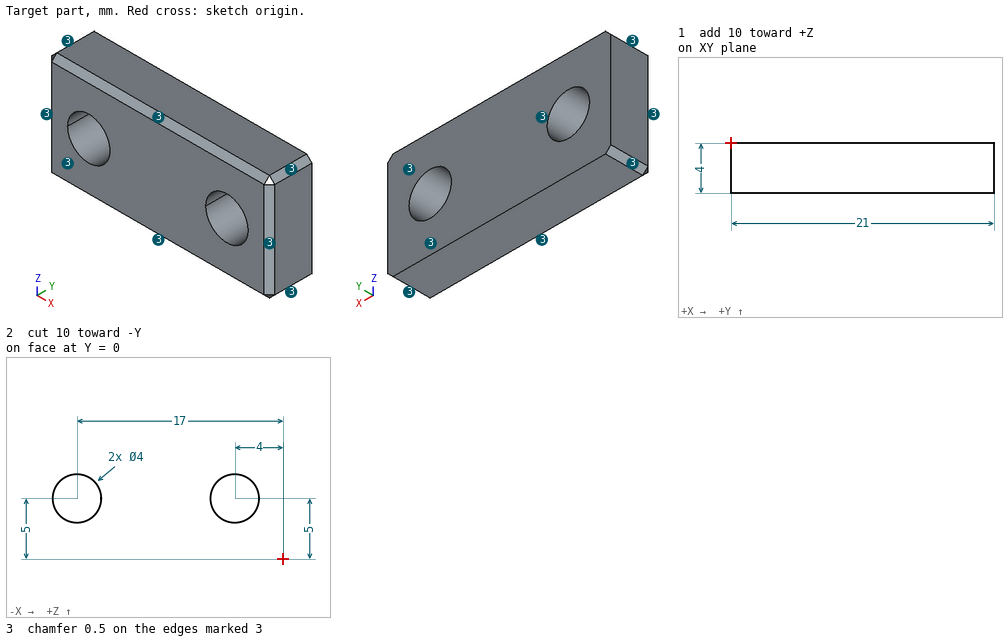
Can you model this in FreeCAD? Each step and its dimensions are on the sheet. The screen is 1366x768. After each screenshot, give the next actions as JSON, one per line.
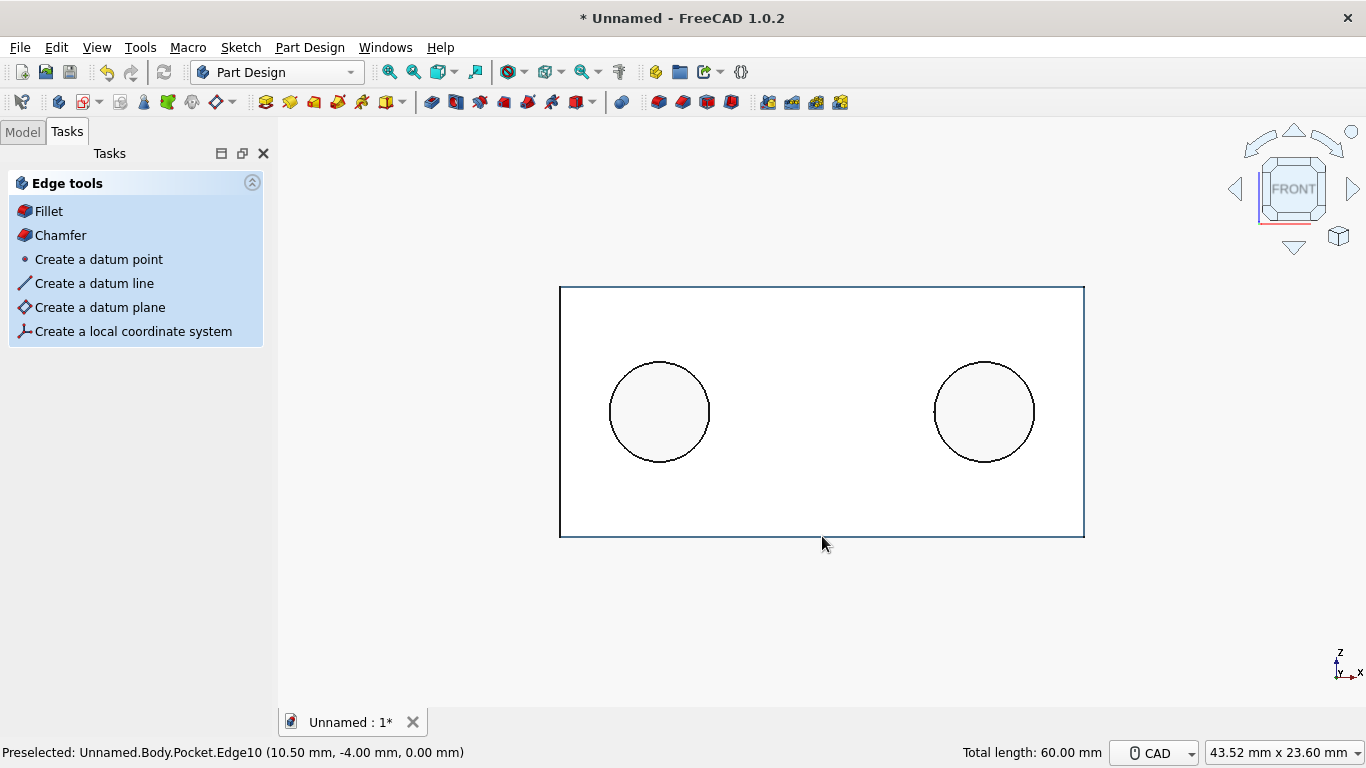
{"action": "left_click", "coordinate": [560, 411], "text": "ctrl"}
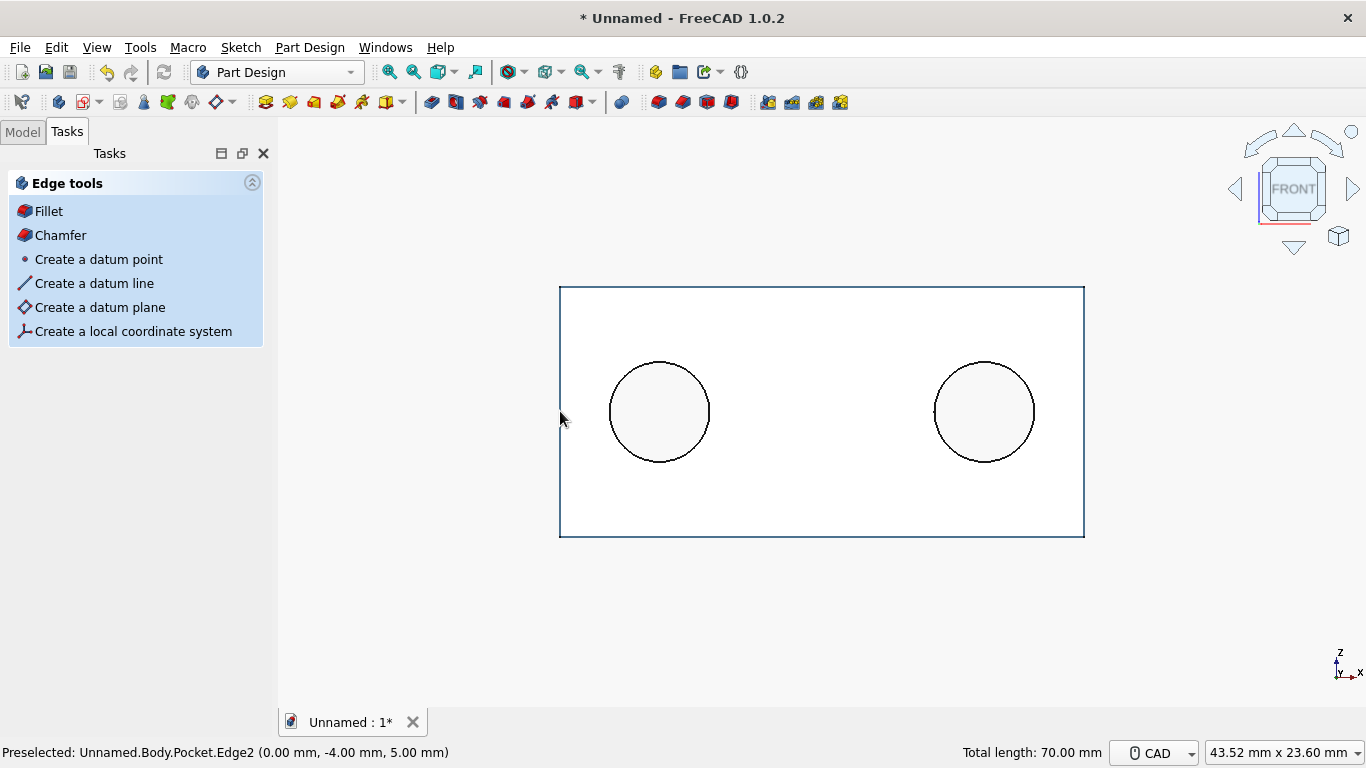
{"action": "key", "text": "3"}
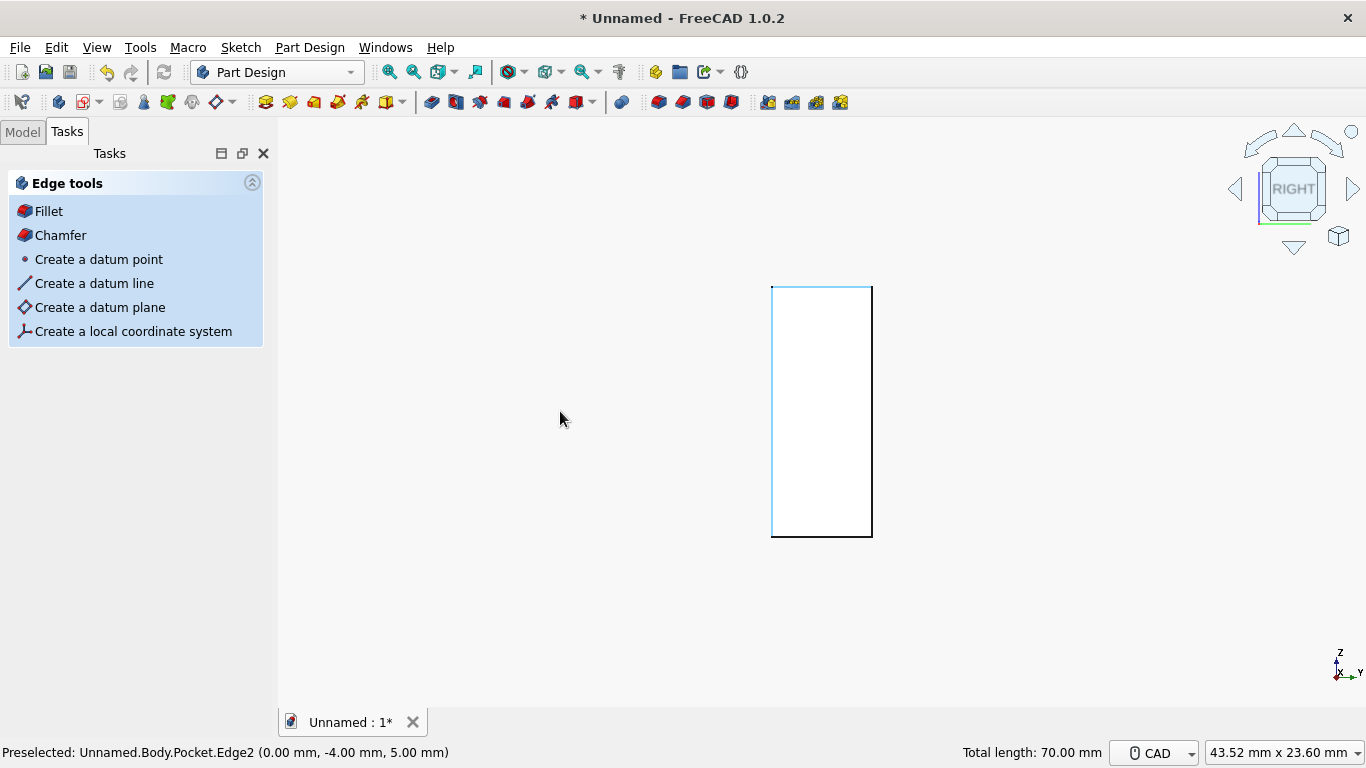
{"action": "left_click", "coordinate": [390, 72]}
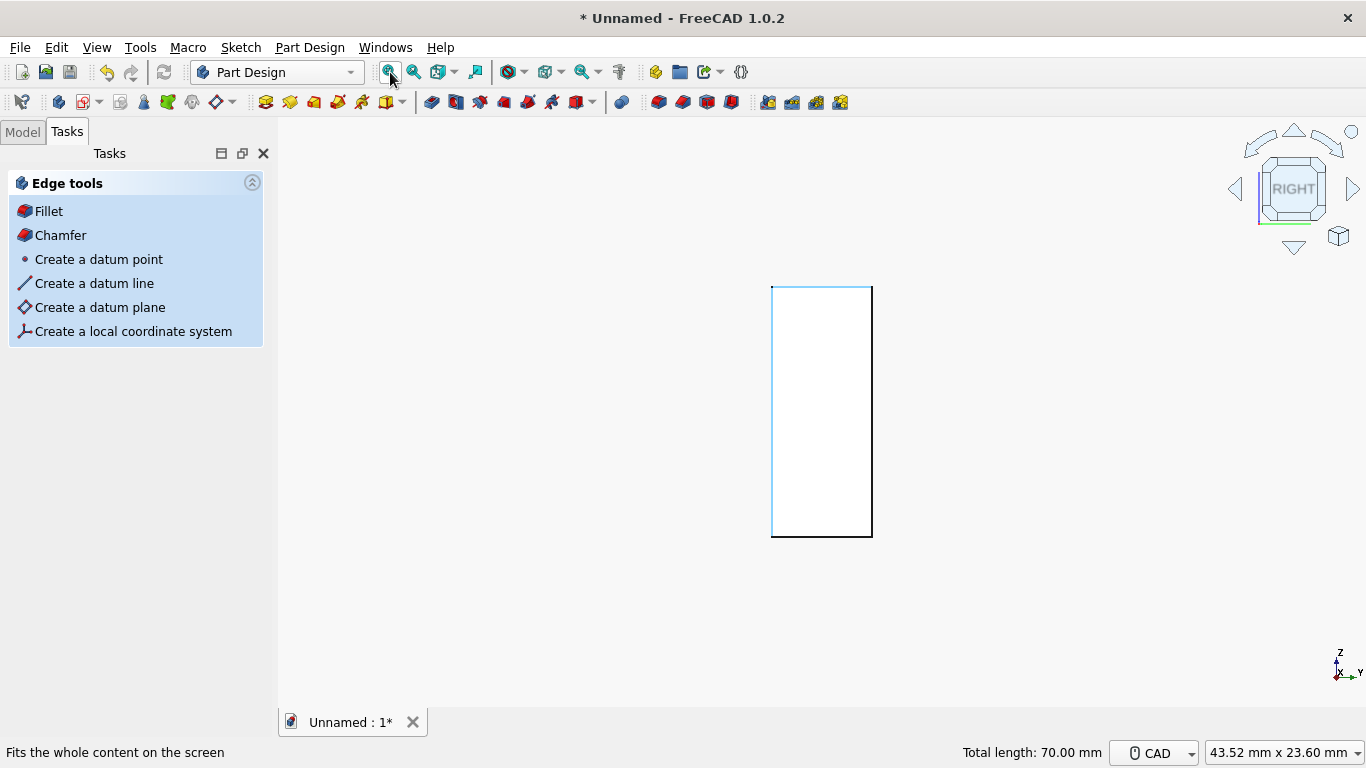
{"action": "left_click", "coordinate": [822, 536], "text": "ctrl"}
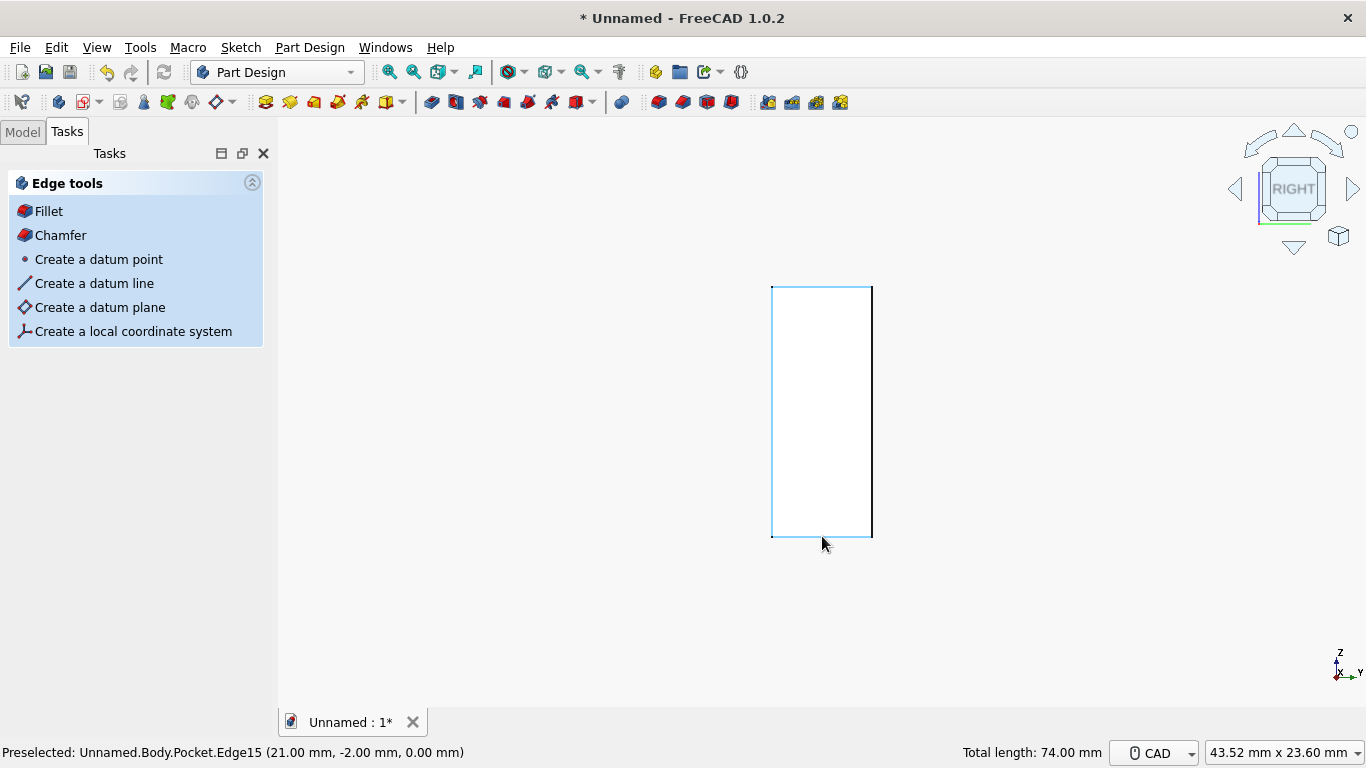
{"action": "key", "text": "5"}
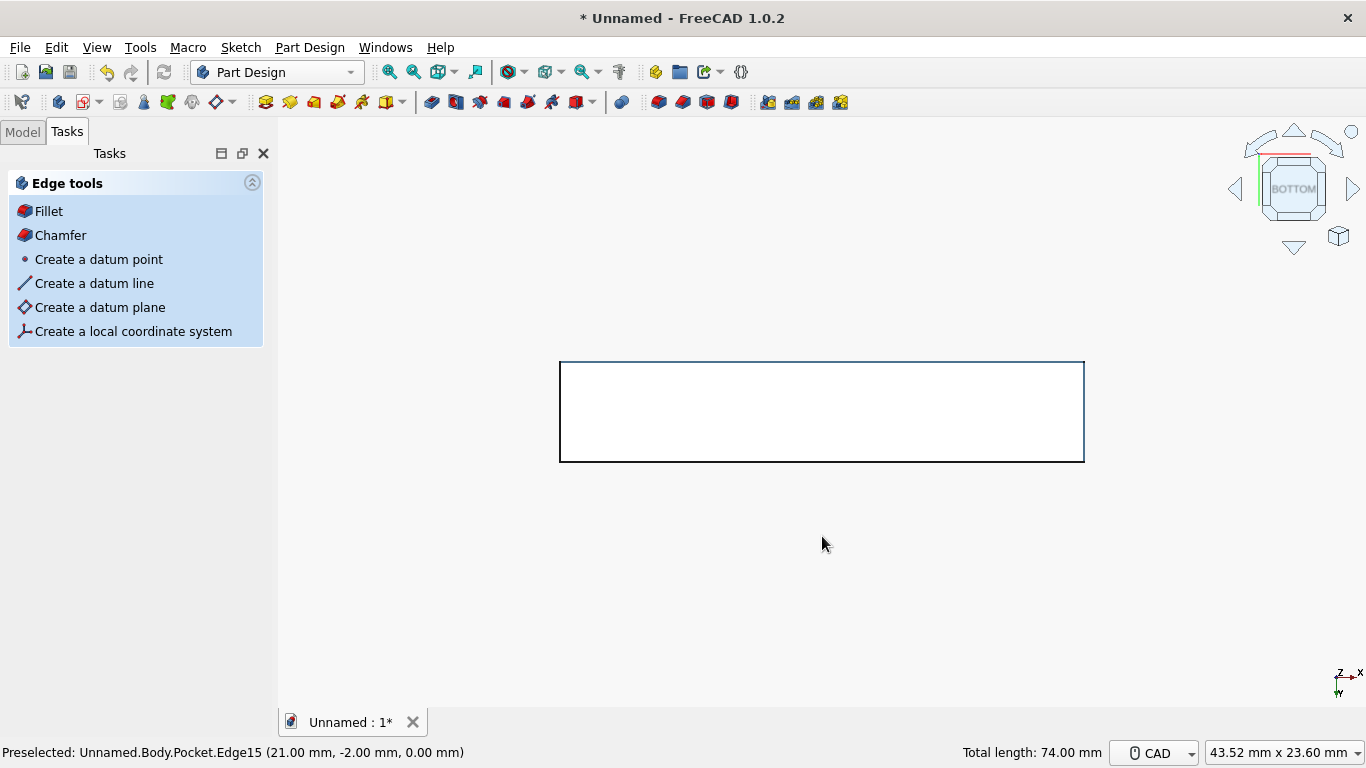
{"action": "left_click", "coordinate": [560, 411], "text": "ctrl"}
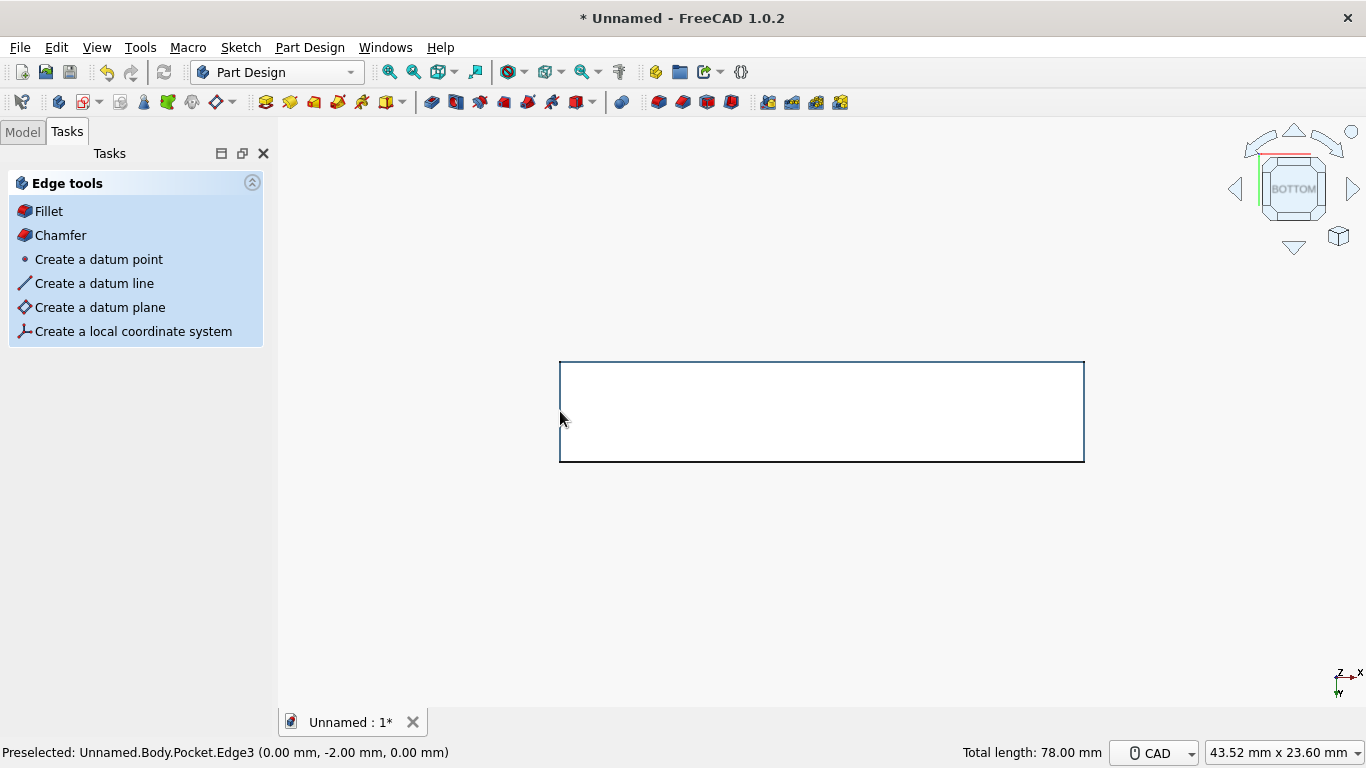
{"action": "left_click", "coordinate": [684, 102]}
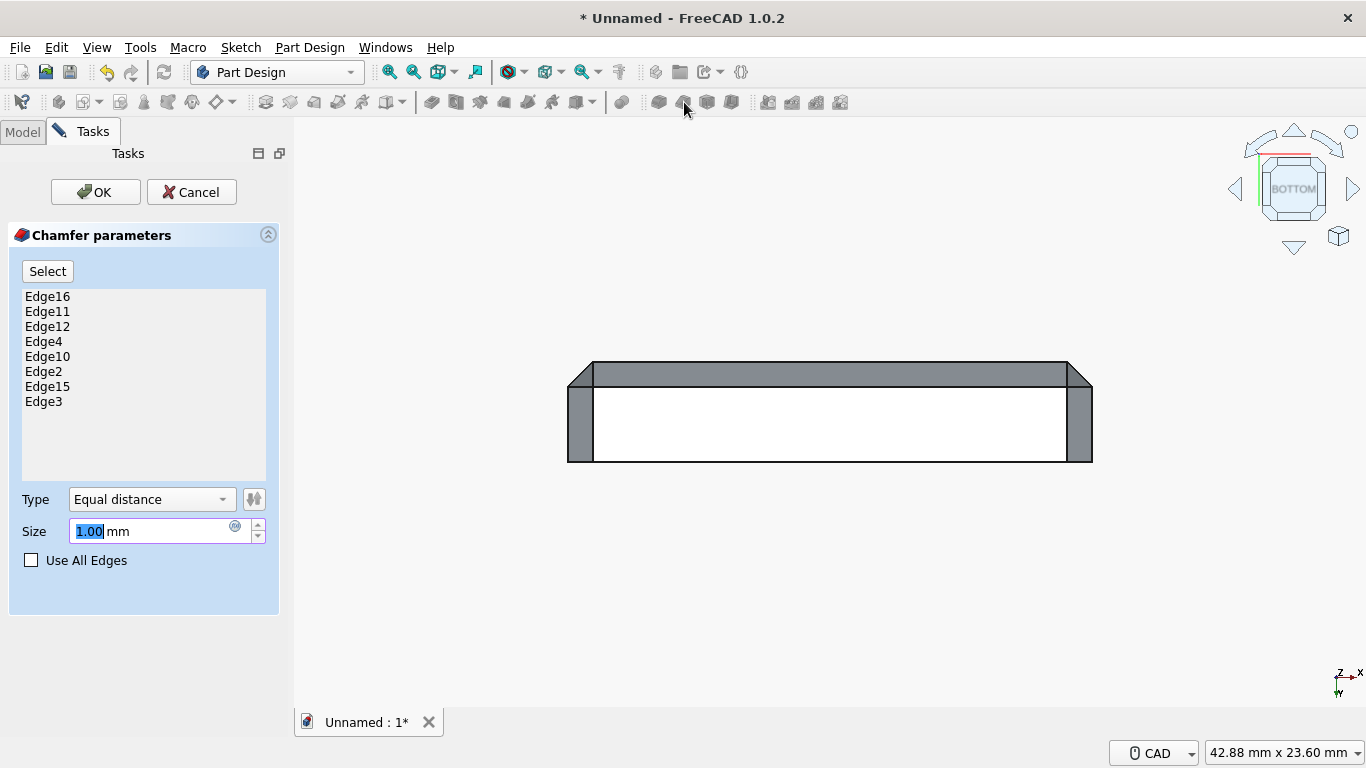
{"action": "type", "text": "0.5"}
{"action": "key", "text": "Tab"}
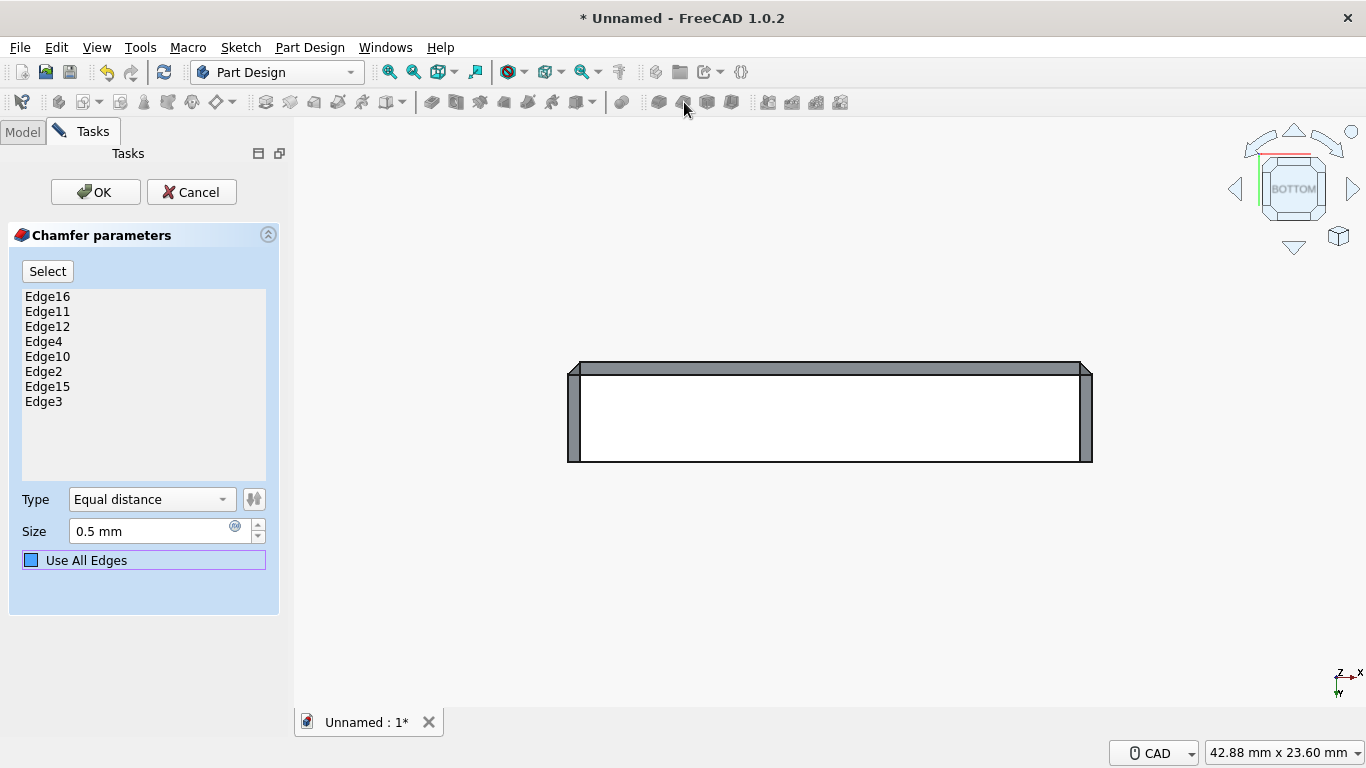
{"action": "left_click", "coordinate": [96, 192]}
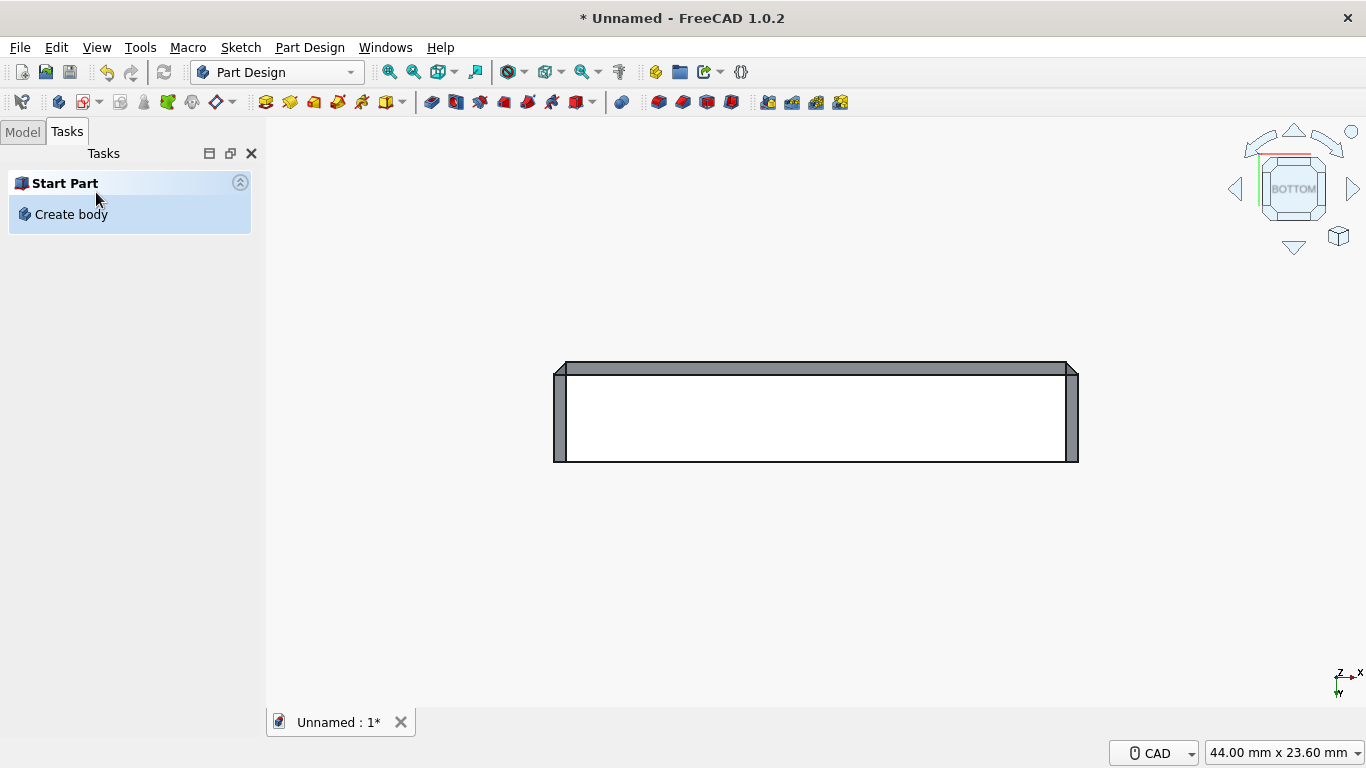
{"action": "key", "text": "0"}